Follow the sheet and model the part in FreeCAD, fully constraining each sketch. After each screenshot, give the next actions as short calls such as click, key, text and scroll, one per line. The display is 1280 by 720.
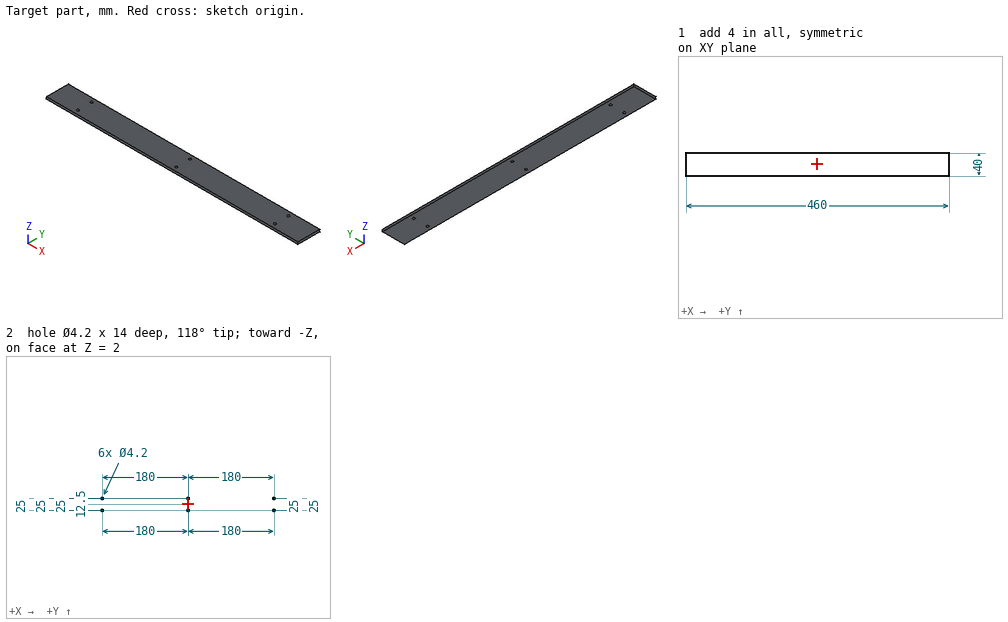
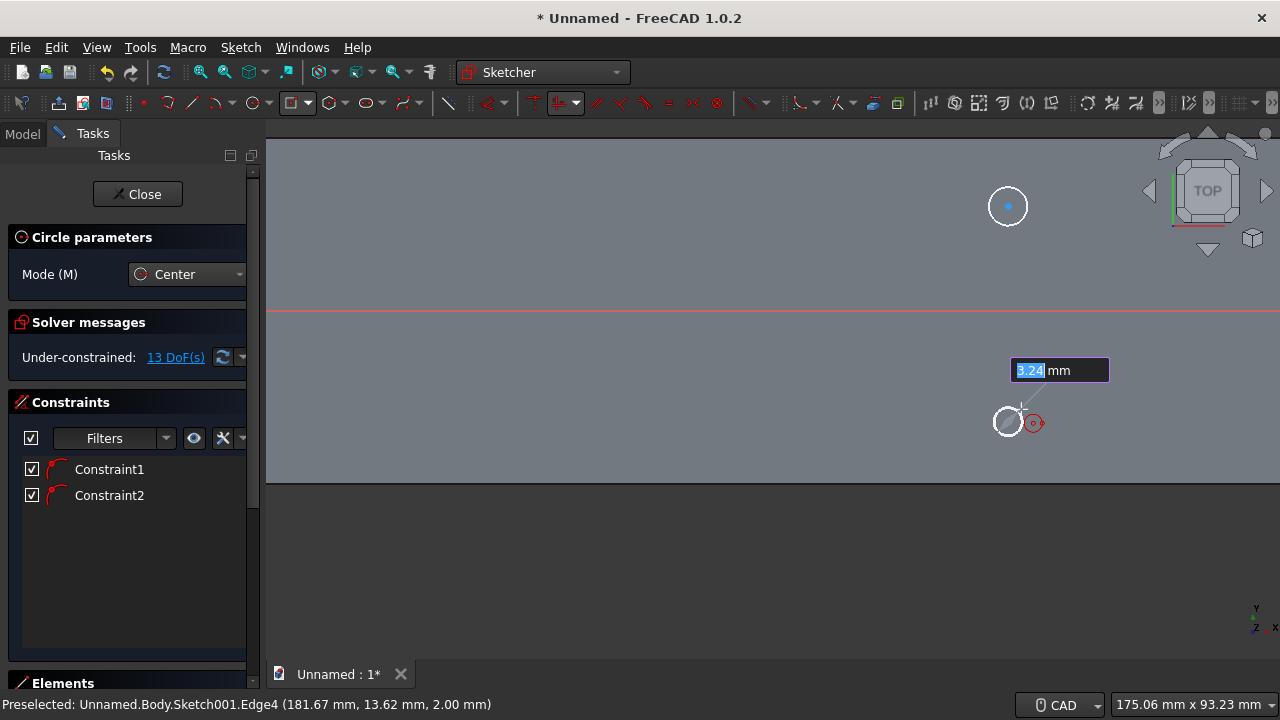
click(1020, 406)
key(Escape)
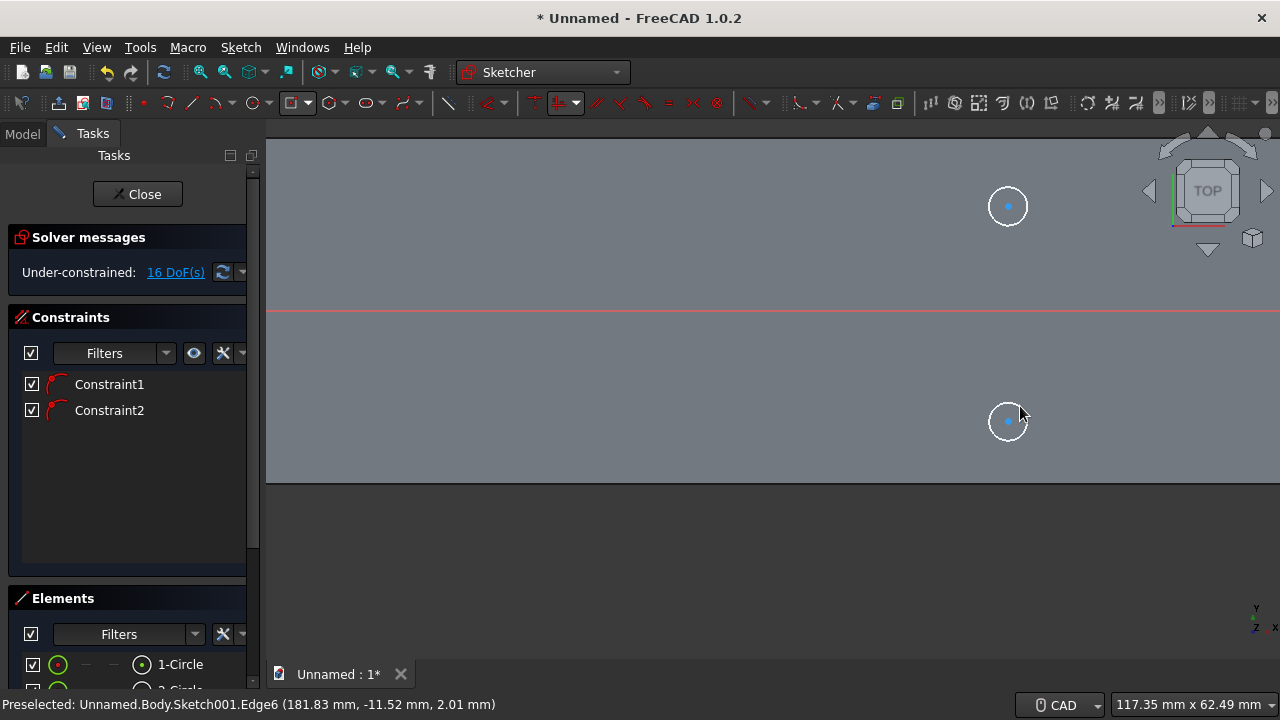
scroll(1021, 409, down, 8)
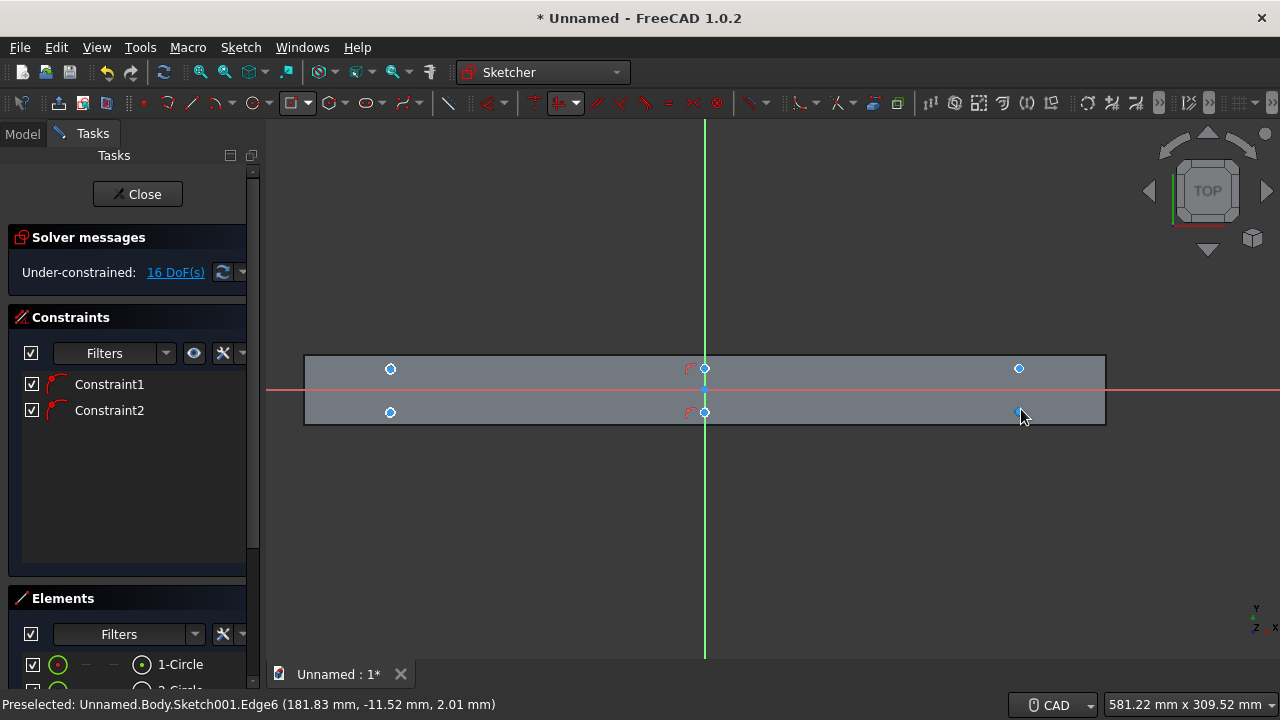
scroll(394, 366, up, 6)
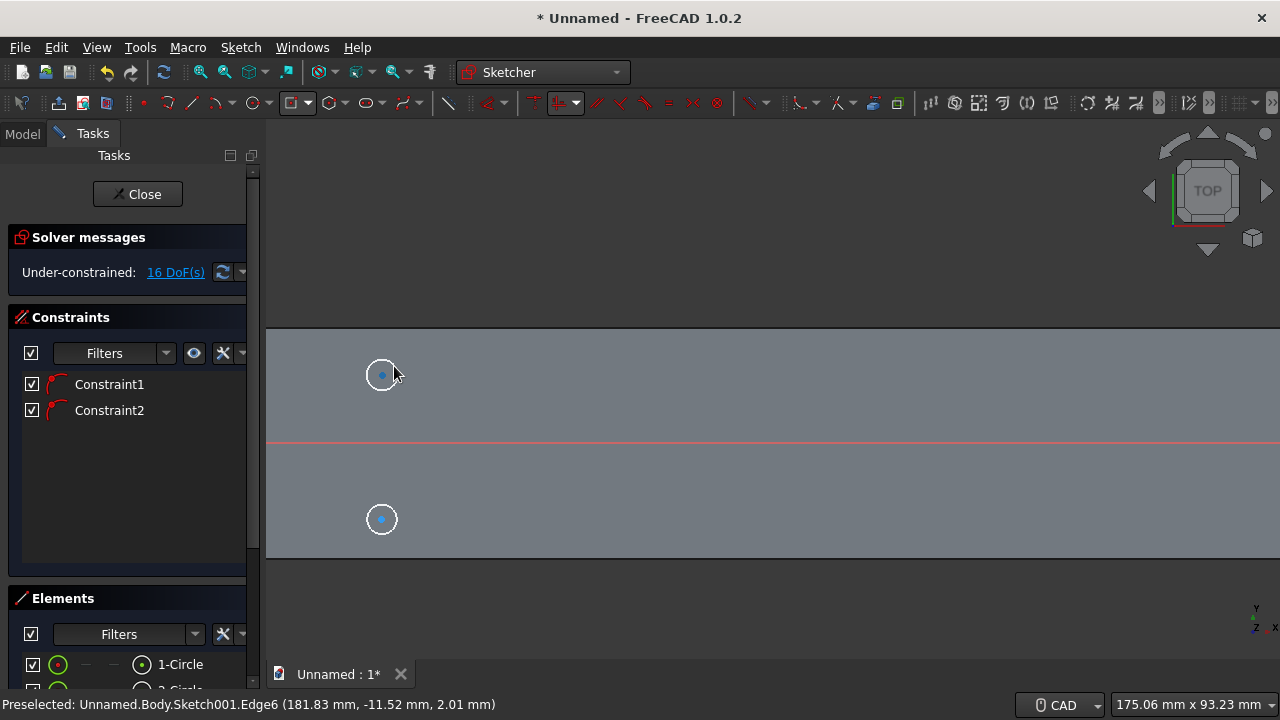
click(393, 364)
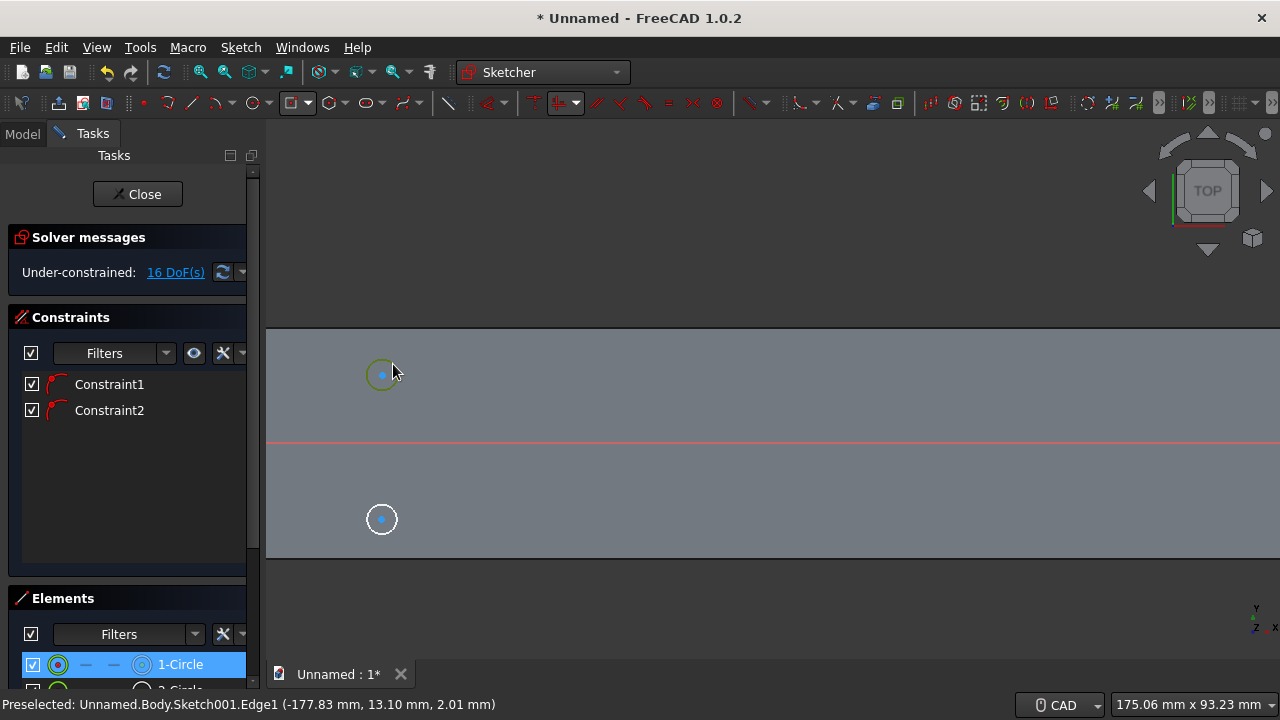
click(392, 509)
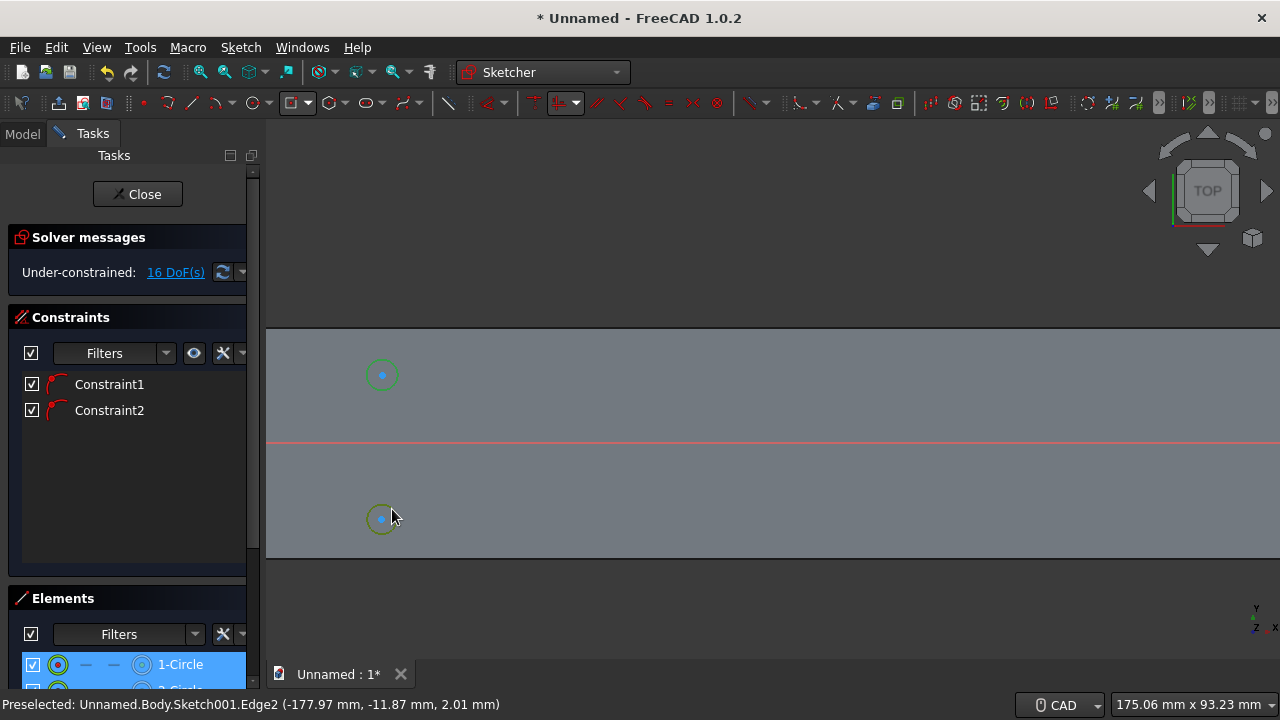
scroll(394, 366, down, 6)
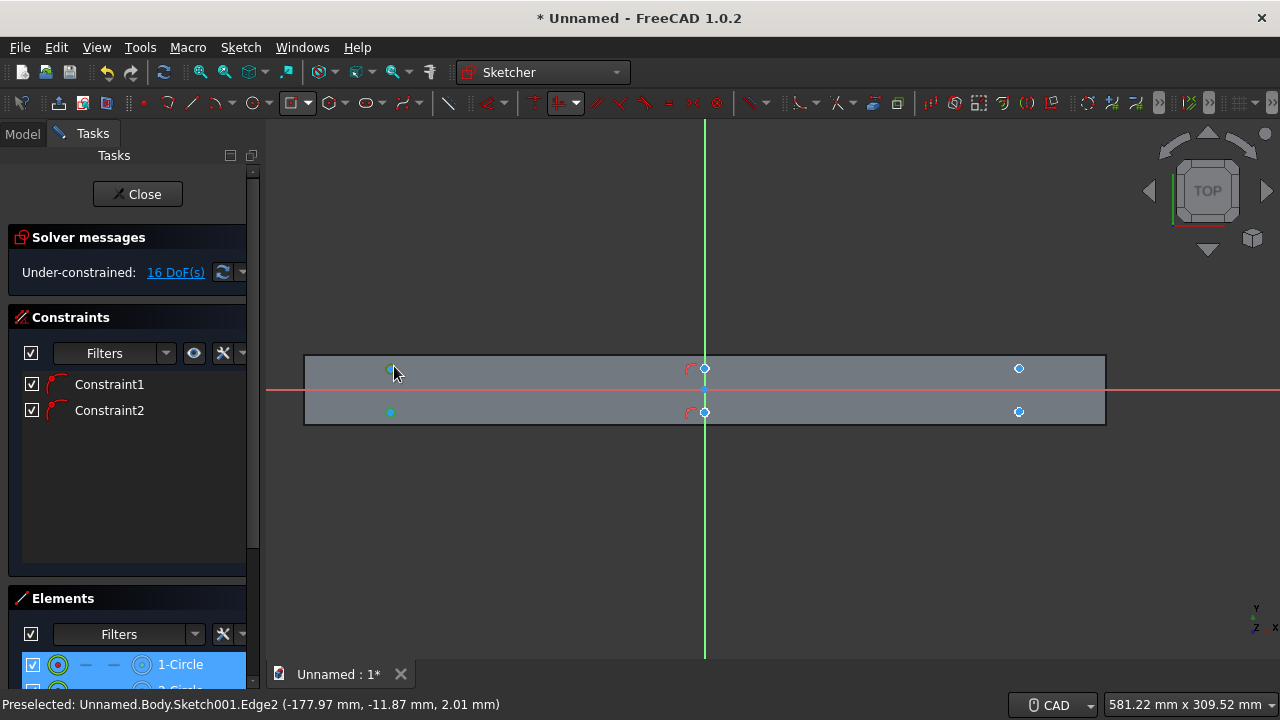
scroll(708, 366, up, 9)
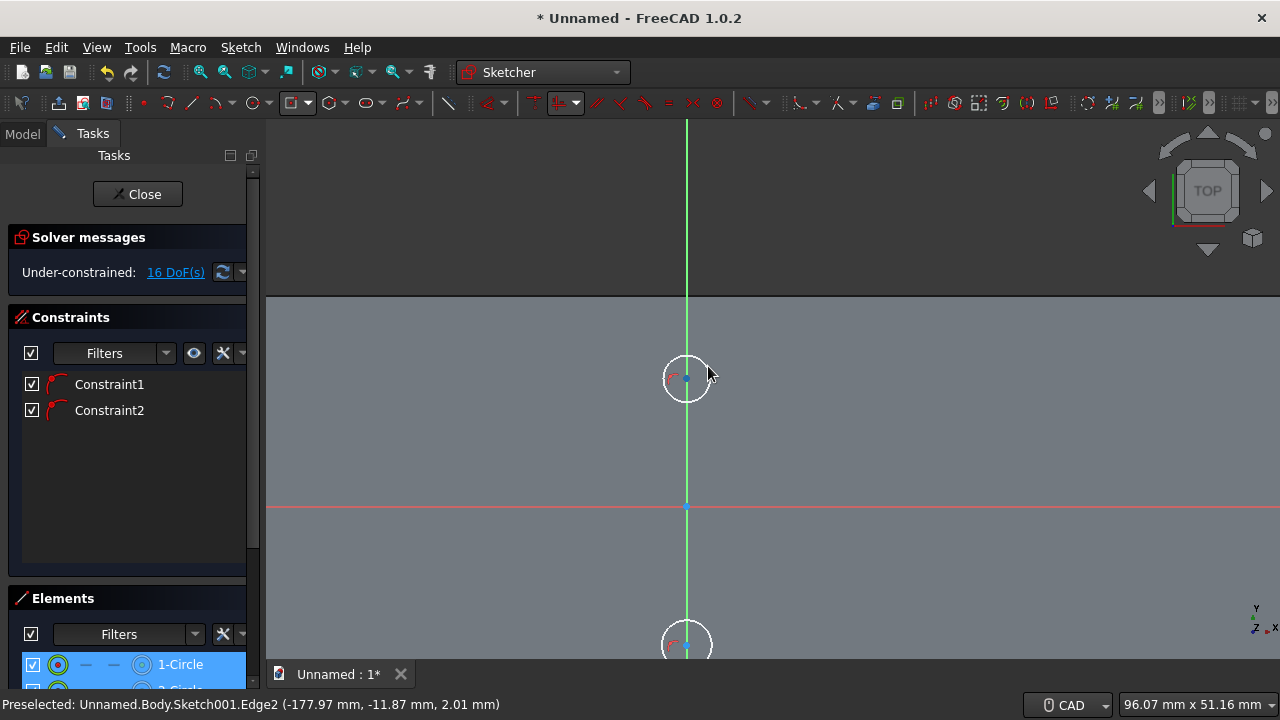
click(703, 362)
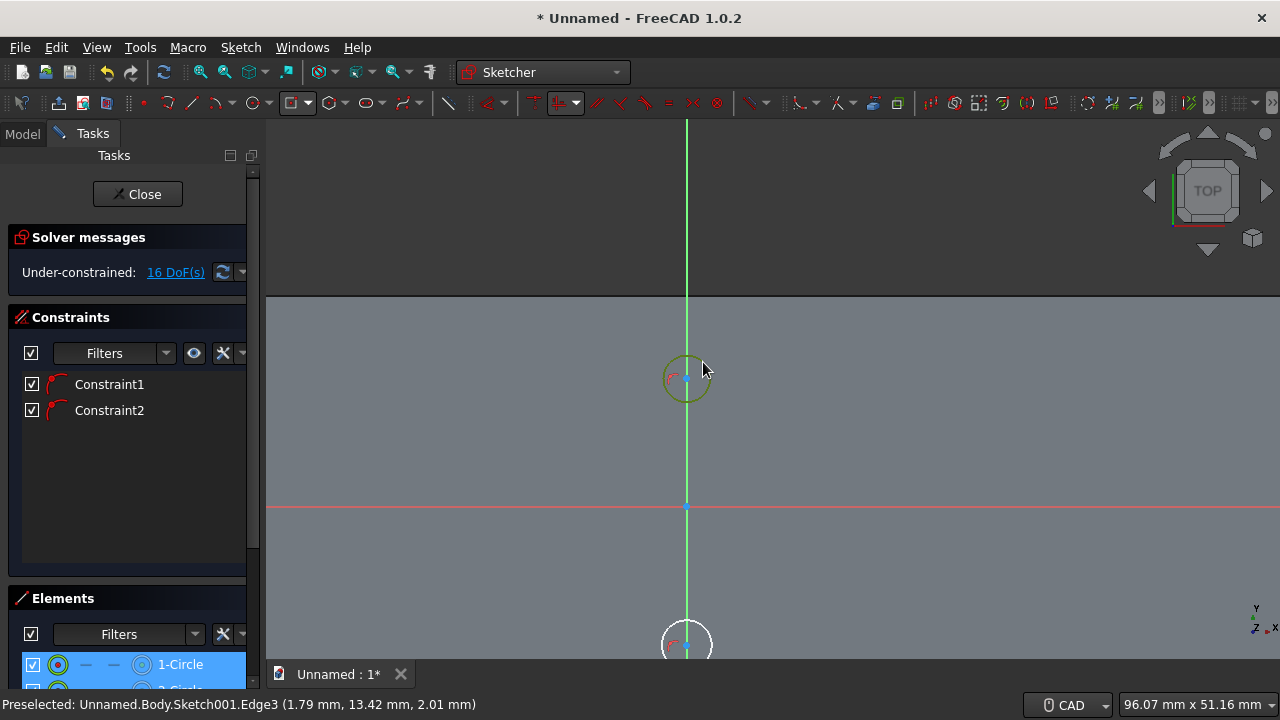
click(704, 627)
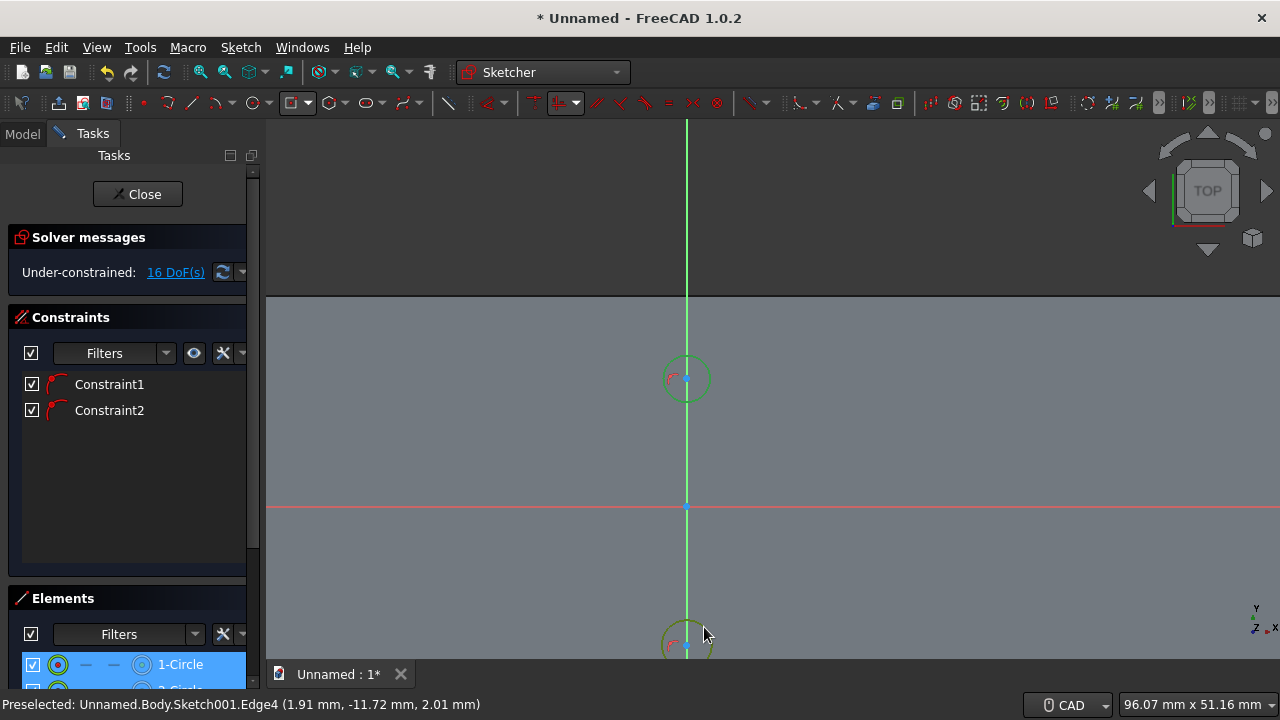
scroll(708, 366, down, 9)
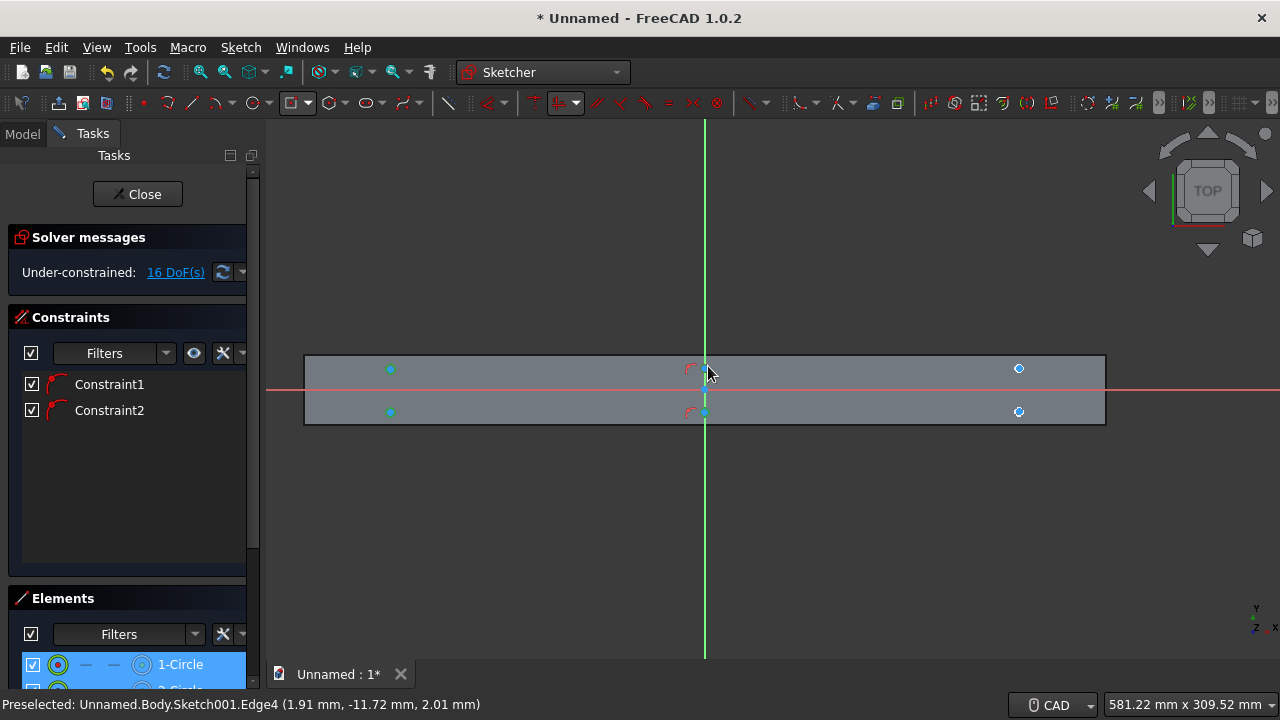
scroll(1022, 366, up, 7)